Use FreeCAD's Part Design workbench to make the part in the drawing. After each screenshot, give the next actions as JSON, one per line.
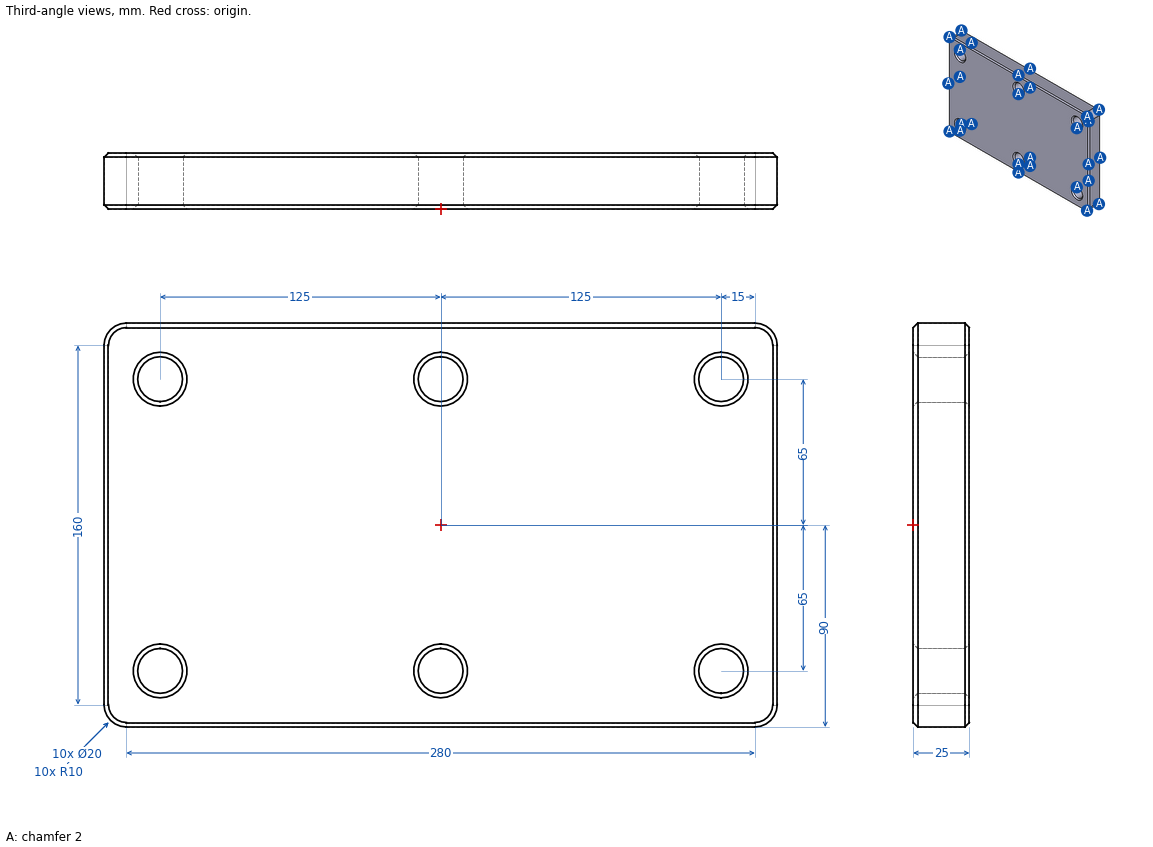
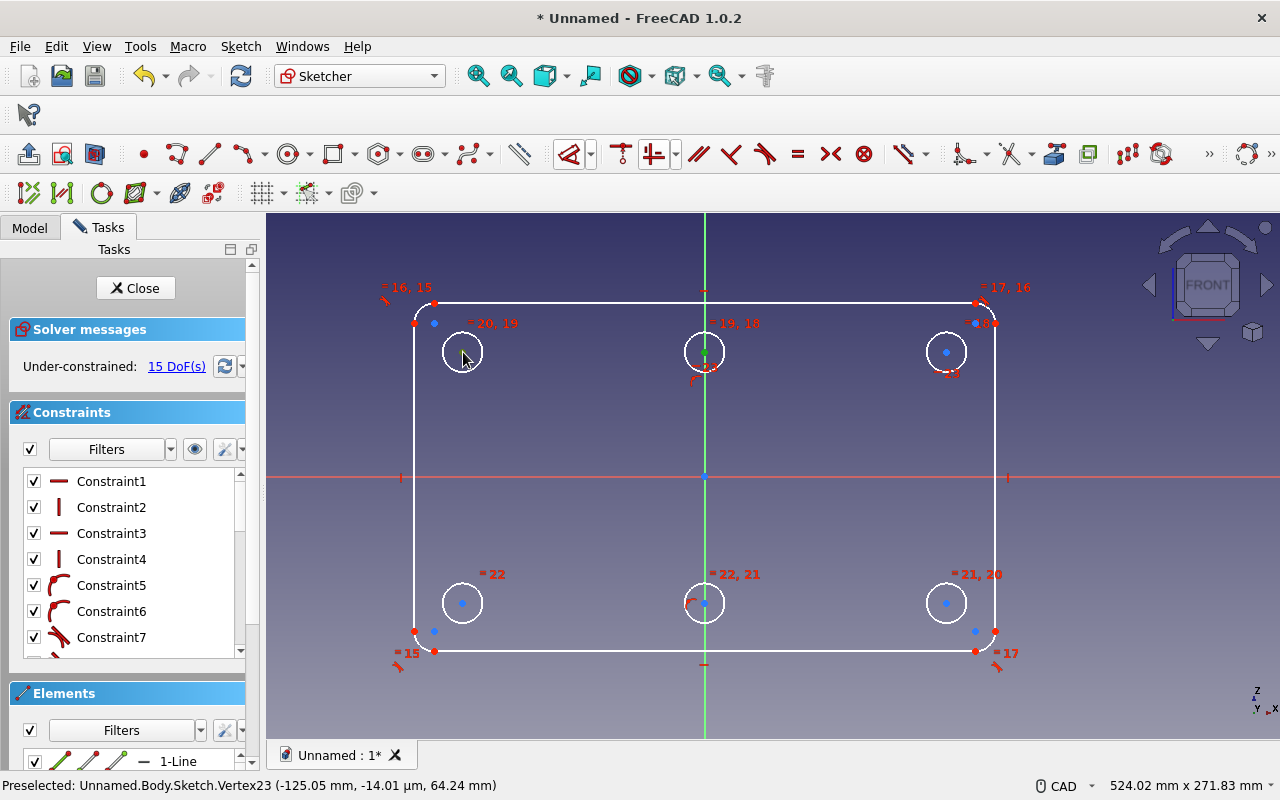
{"action": "left_click", "coordinate": [676, 154]}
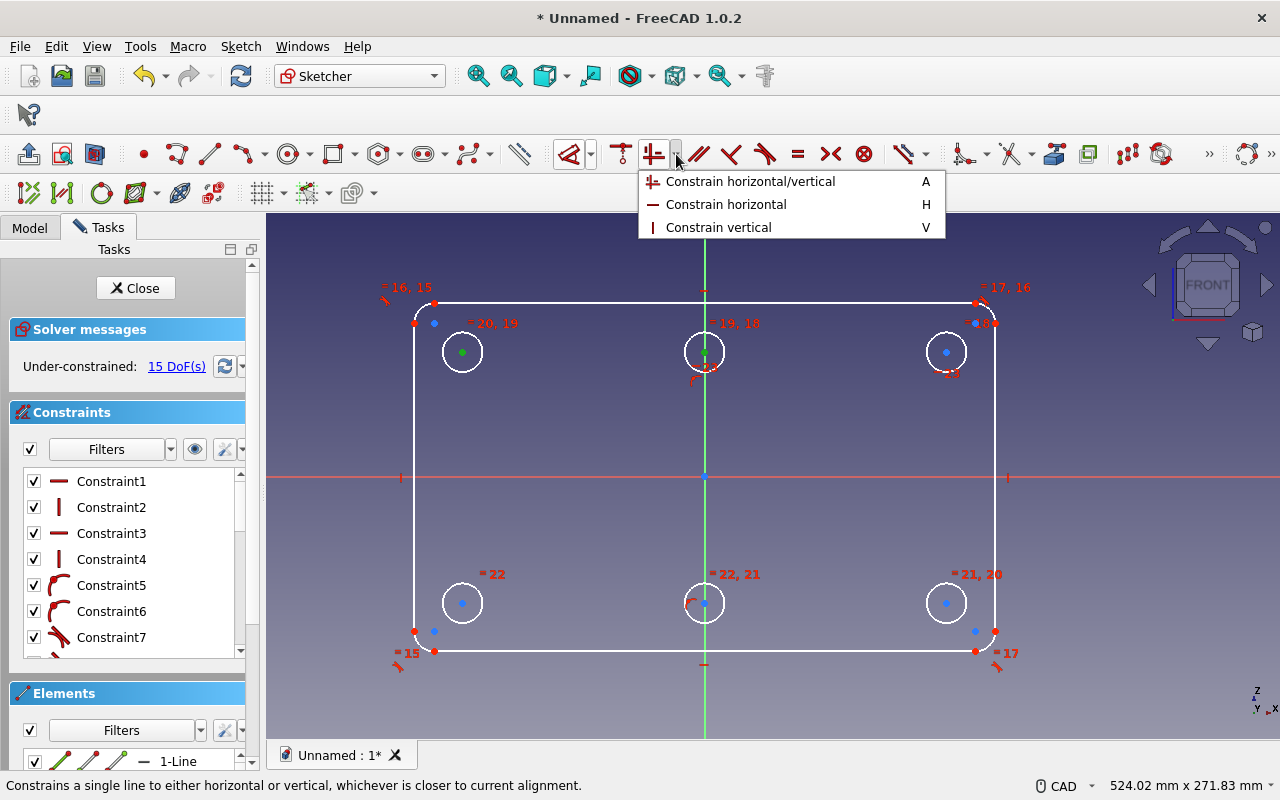
{"action": "left_click", "coordinate": [792, 204]}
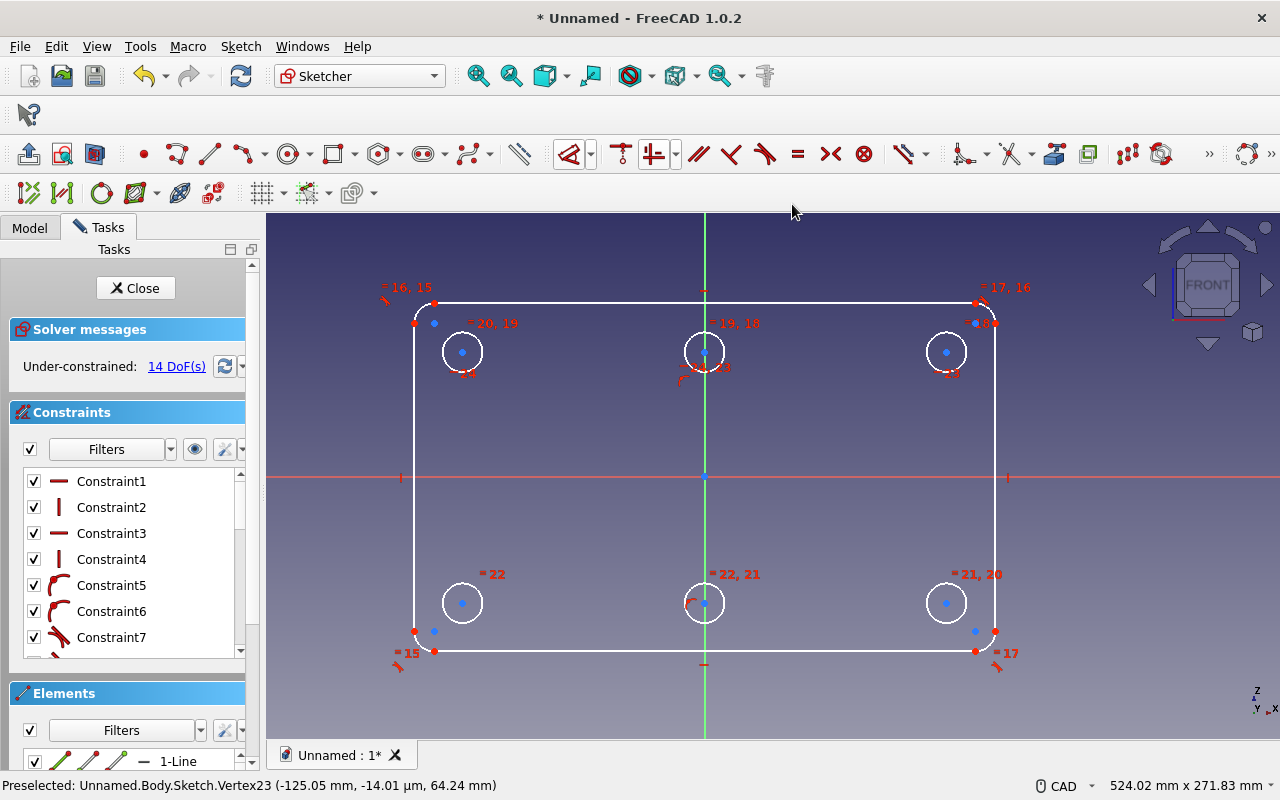
{"action": "left_click", "coordinate": [947, 352]}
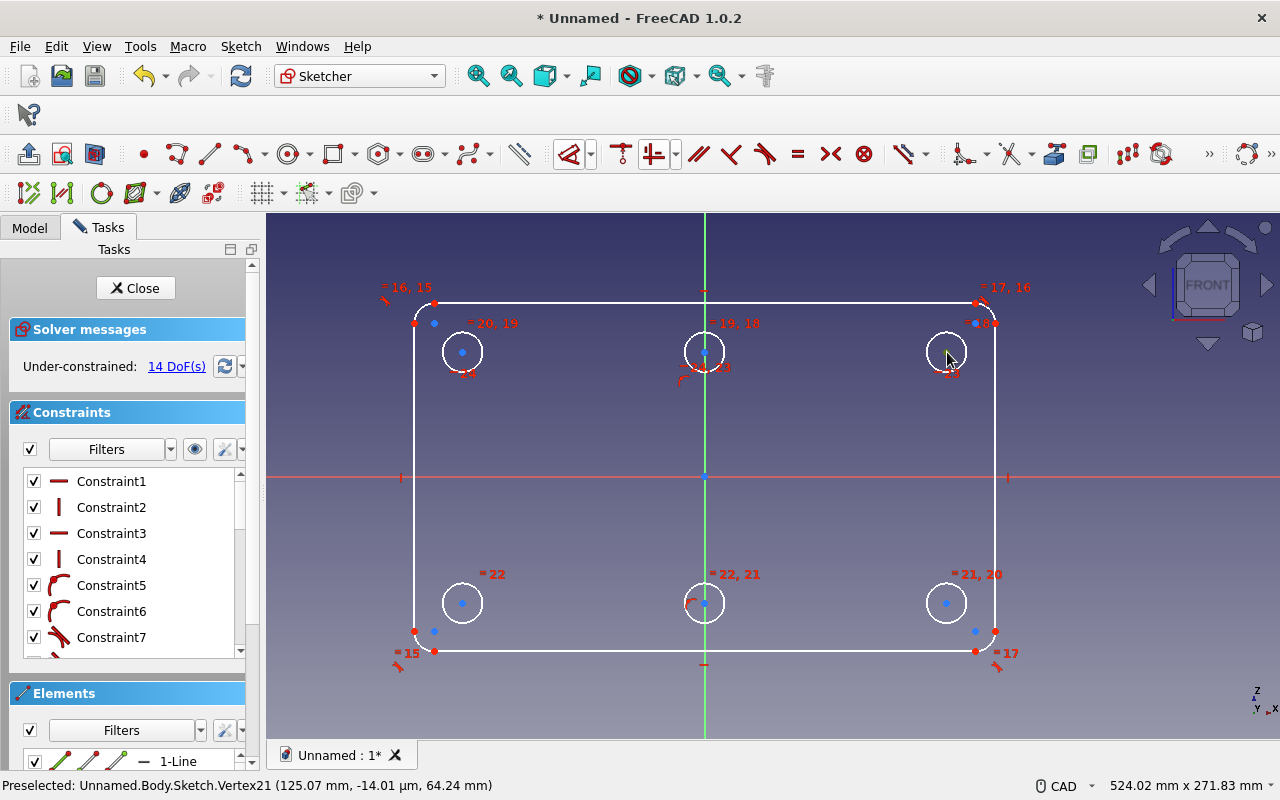
{"action": "left_click", "coordinate": [947, 603]}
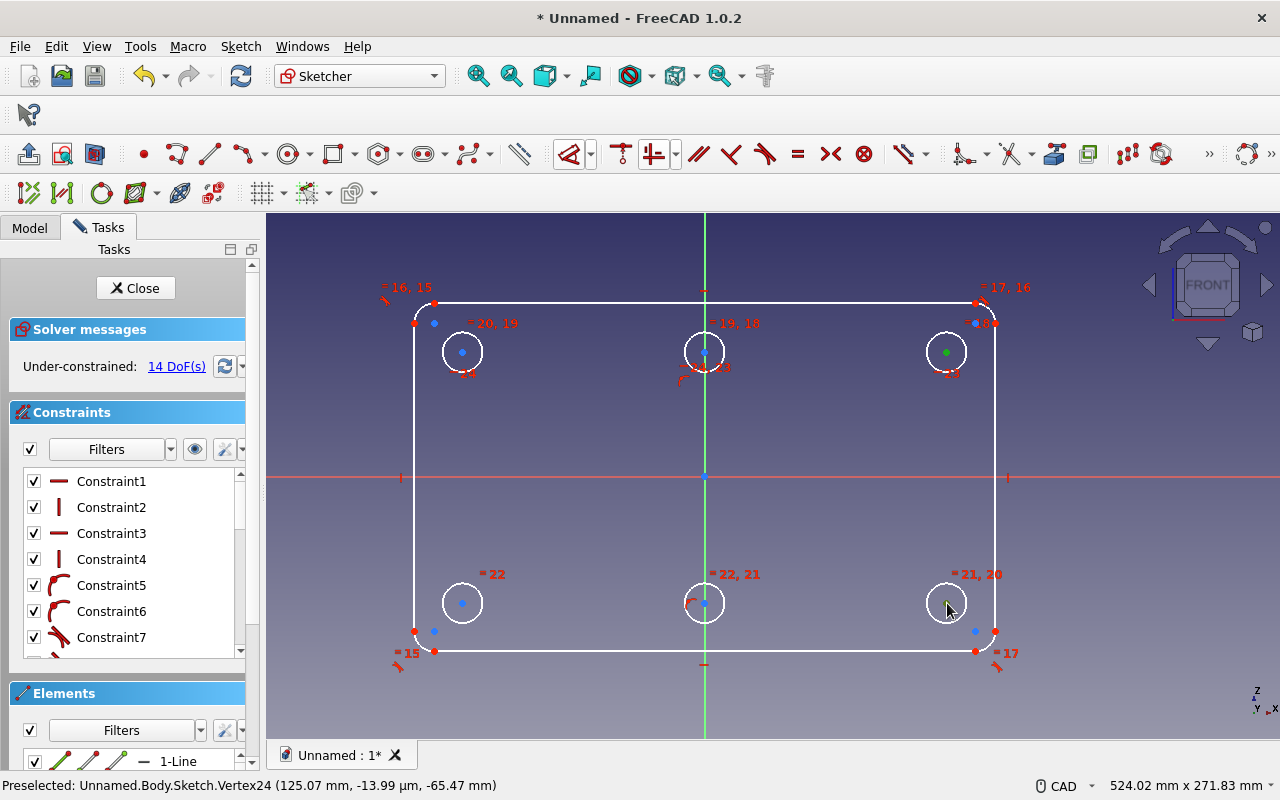
{"action": "left_click", "coordinate": [676, 154]}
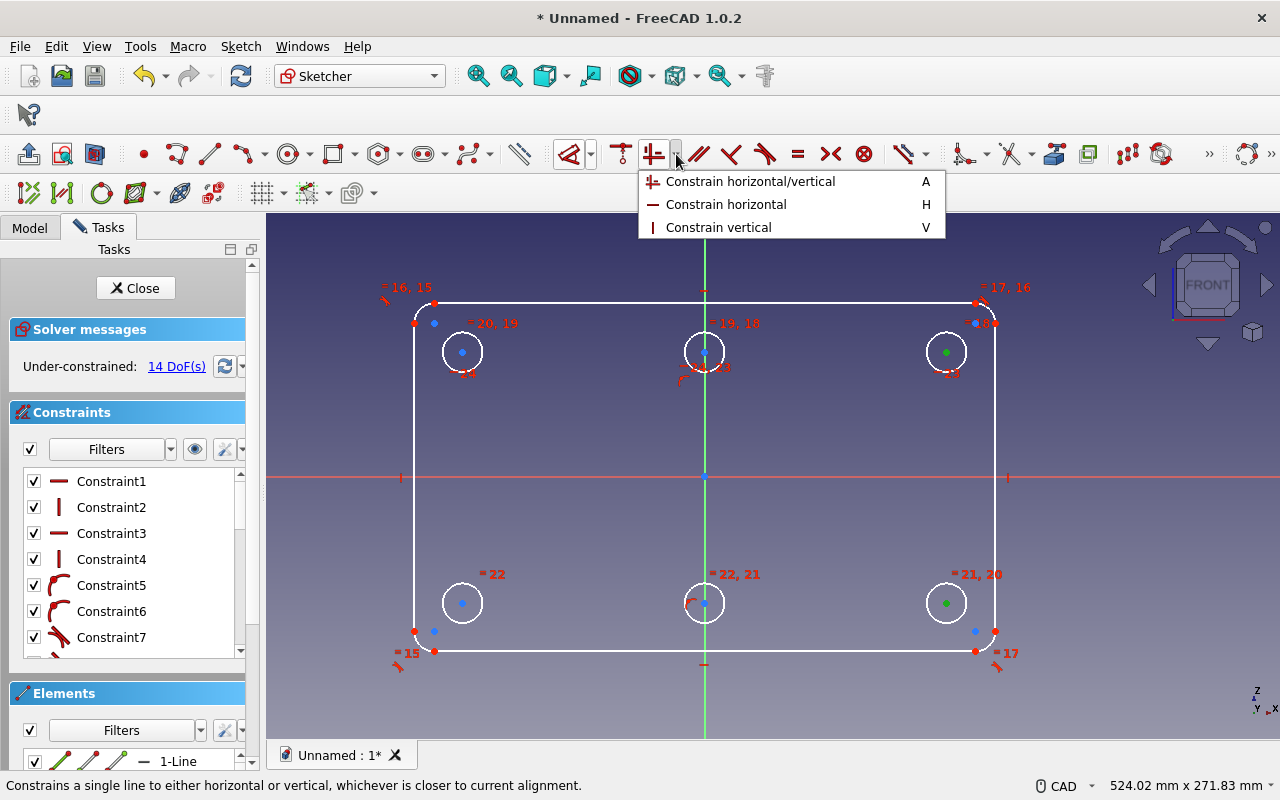
{"action": "left_click", "coordinate": [792, 228]}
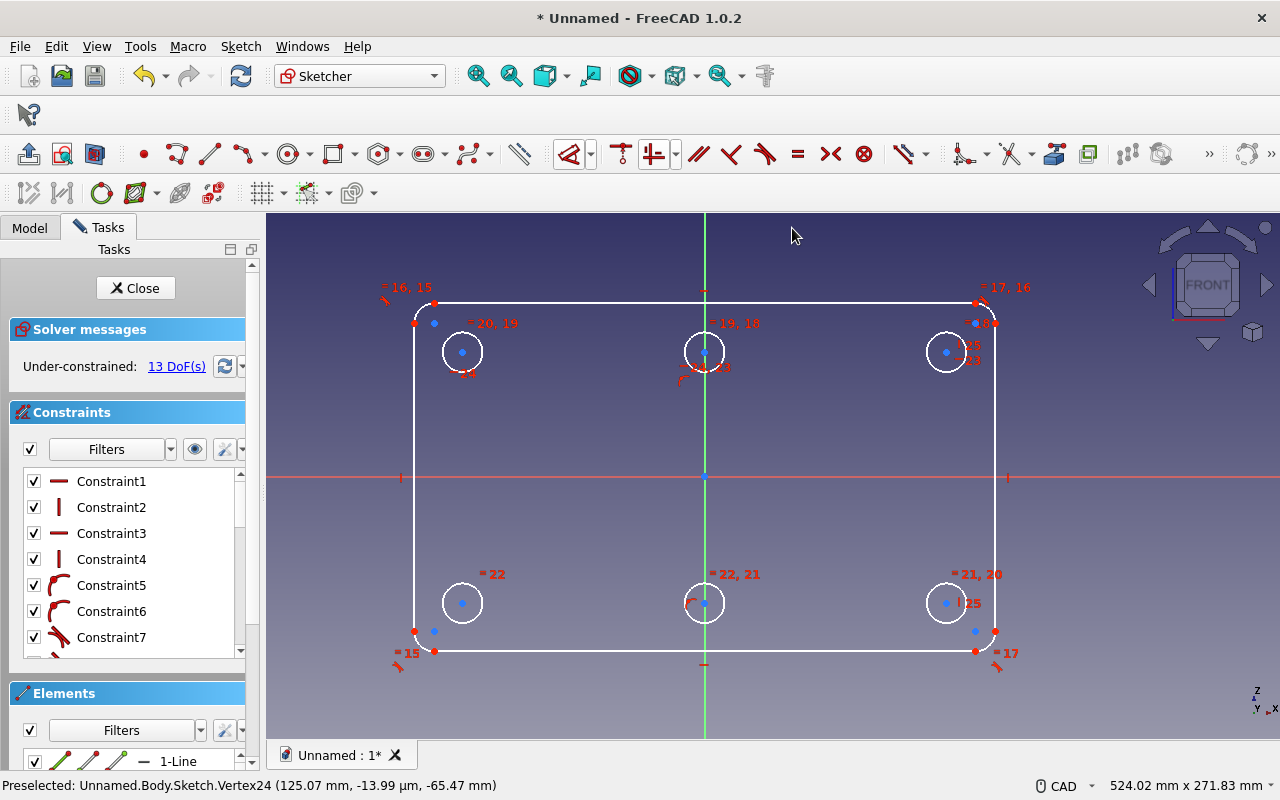
{"action": "left_click", "coordinate": [947, 603]}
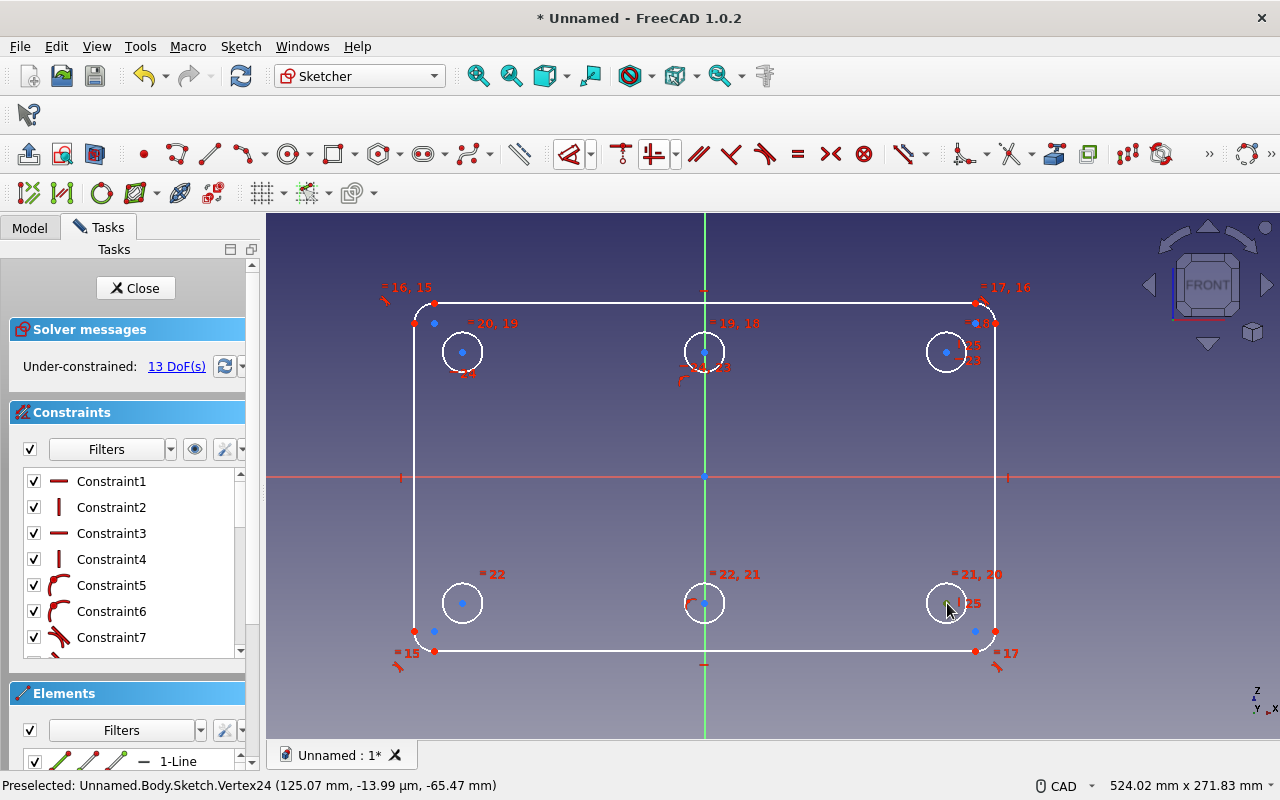
{"action": "left_click", "coordinate": [705, 603]}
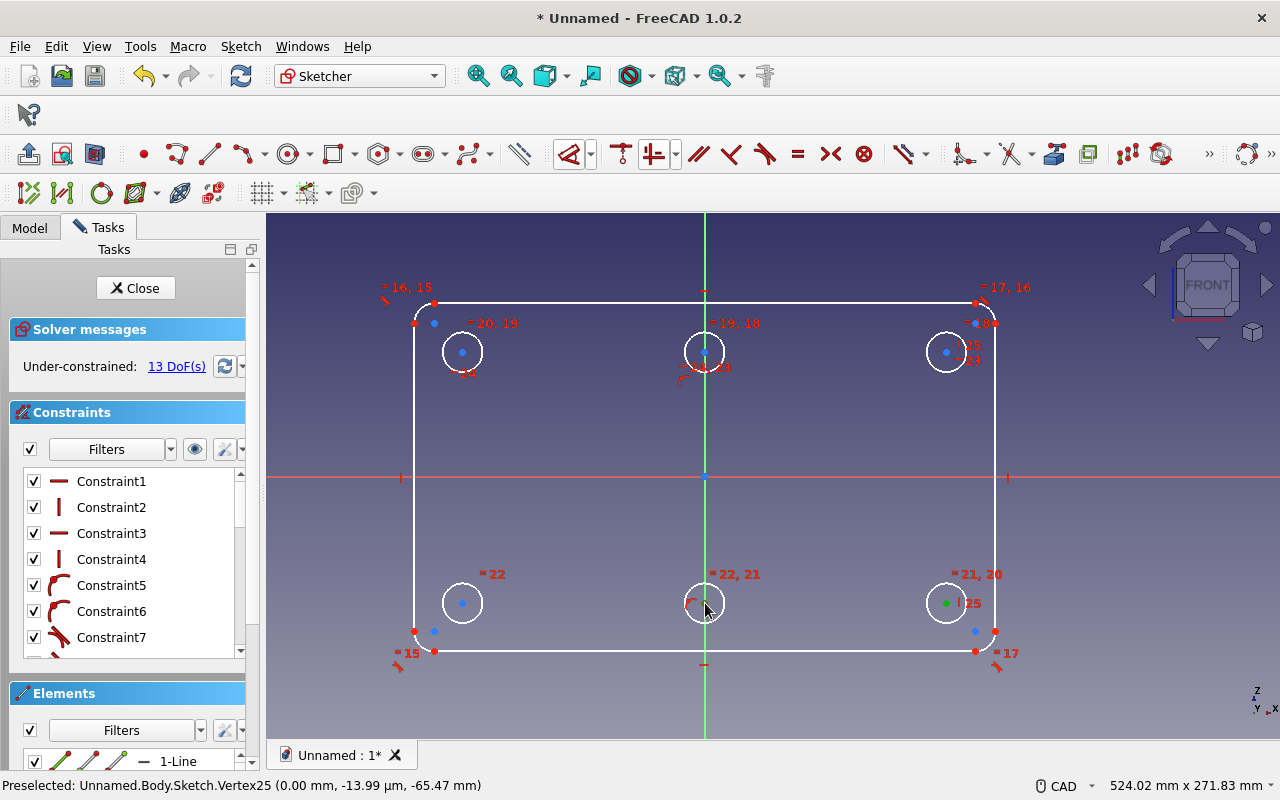
{"action": "left_click", "coordinate": [676, 154]}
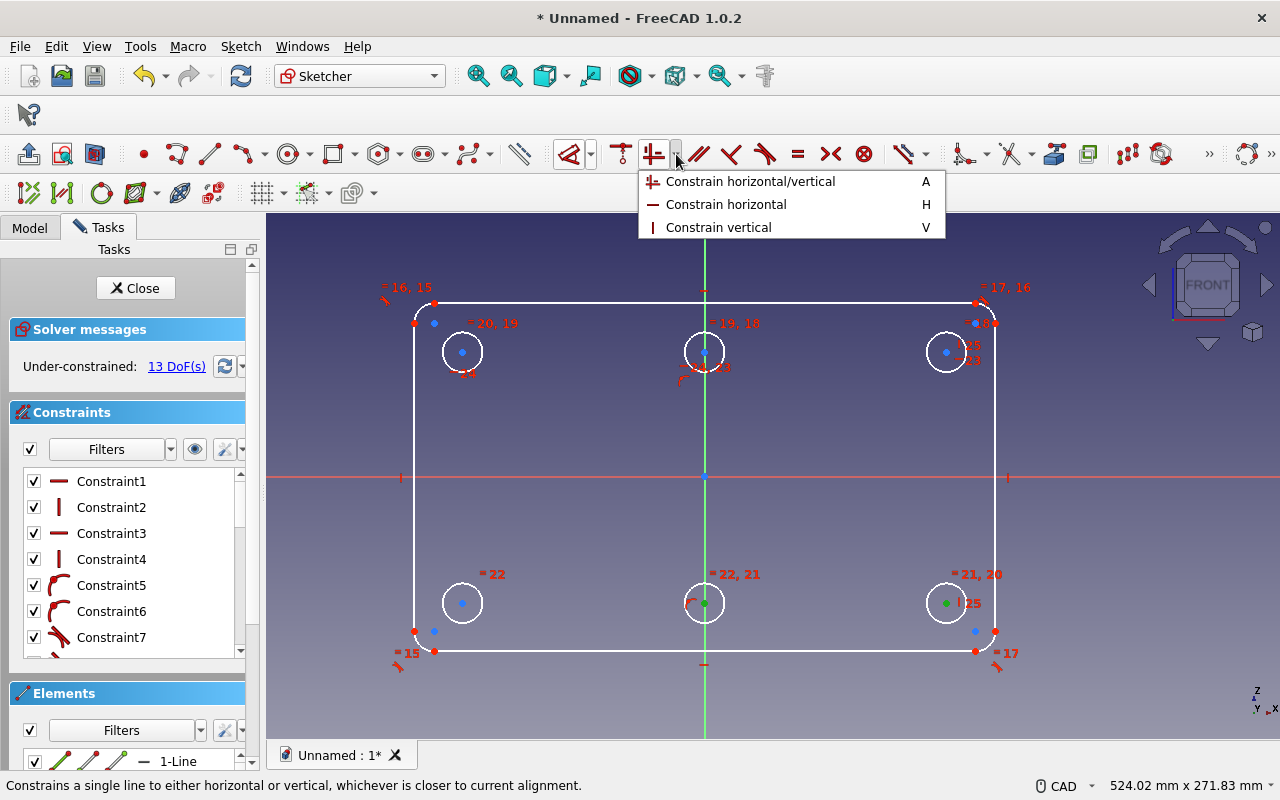
{"action": "left_click", "coordinate": [792, 204]}